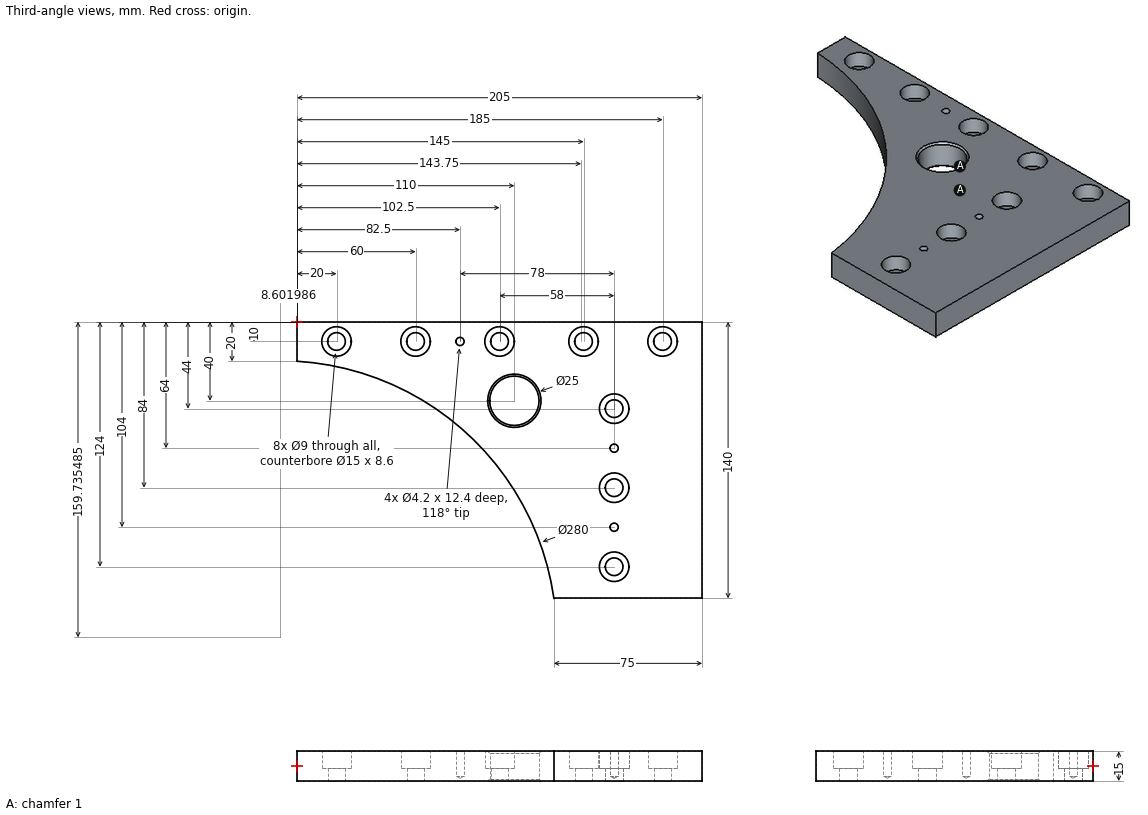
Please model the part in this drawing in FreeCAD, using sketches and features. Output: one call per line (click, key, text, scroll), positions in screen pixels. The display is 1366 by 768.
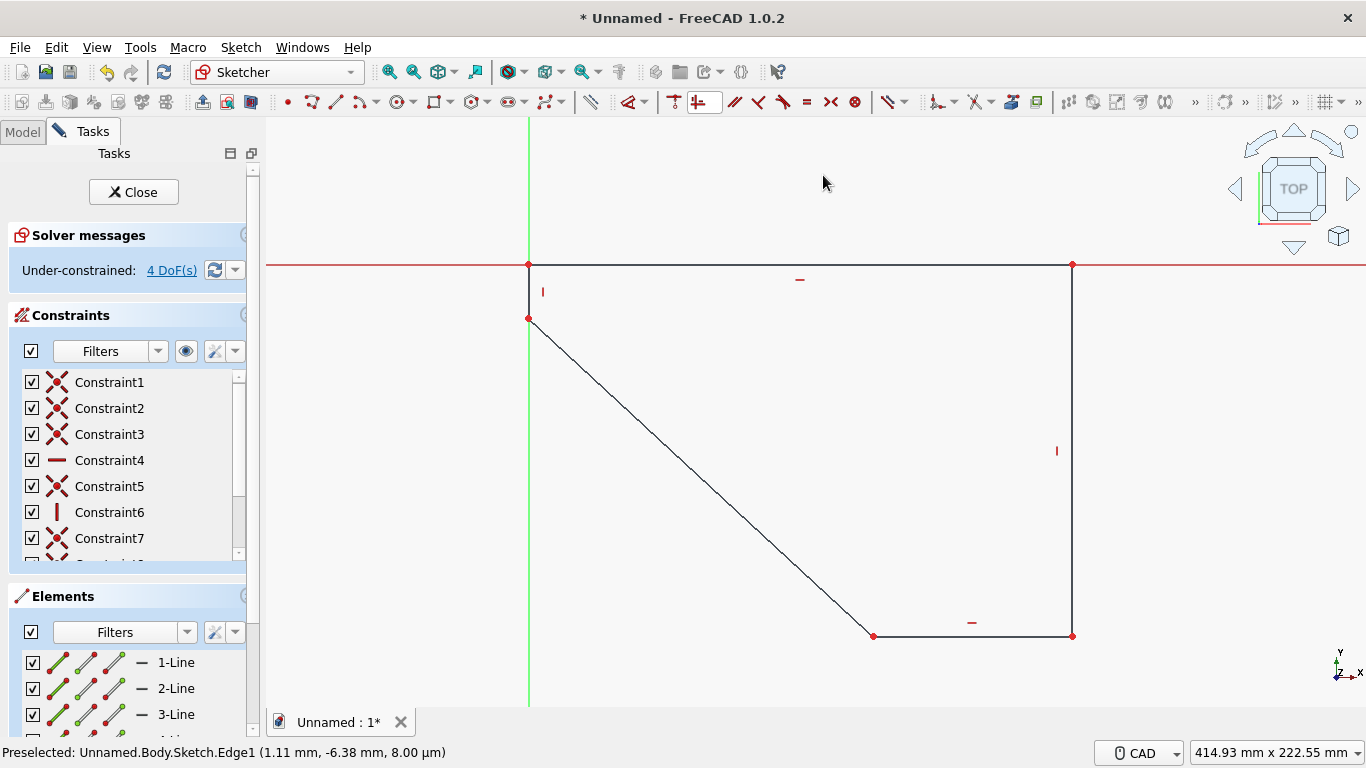
click(529, 281)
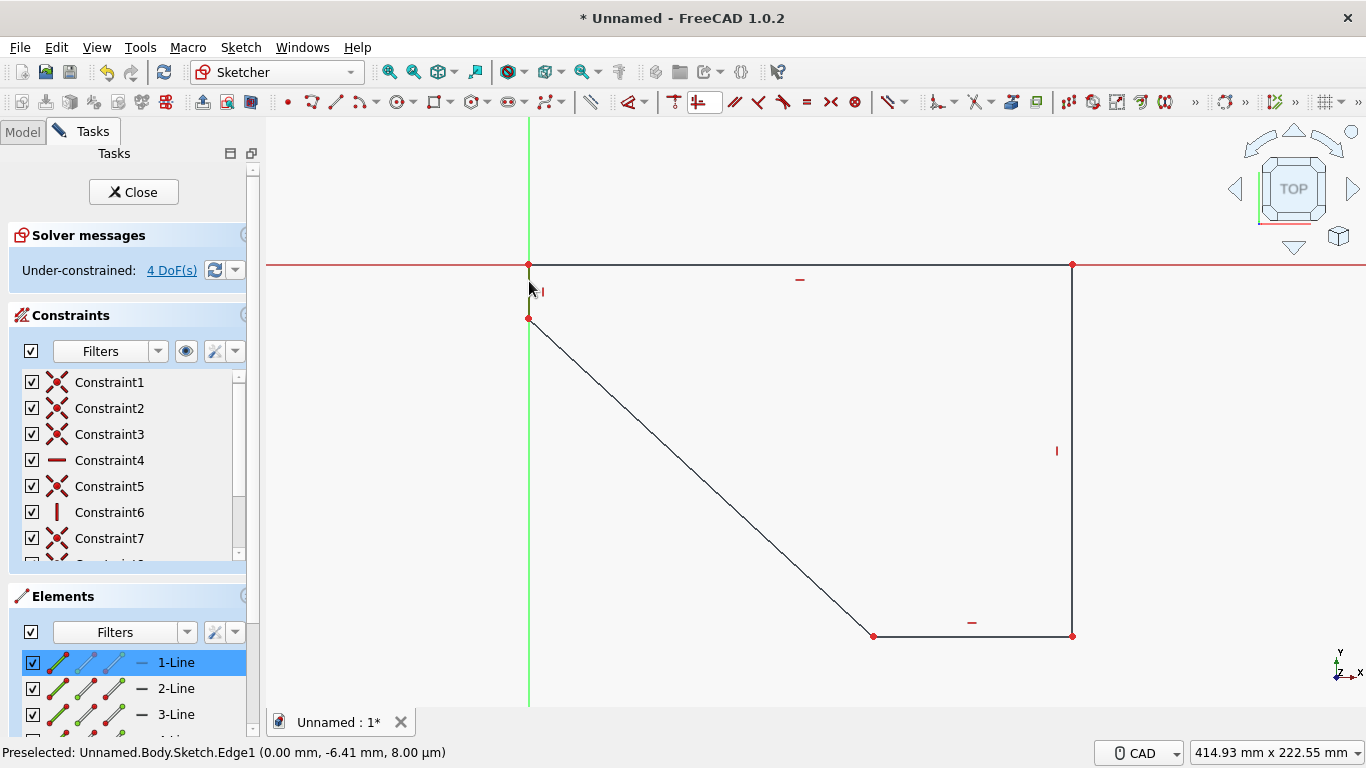
click(646, 102)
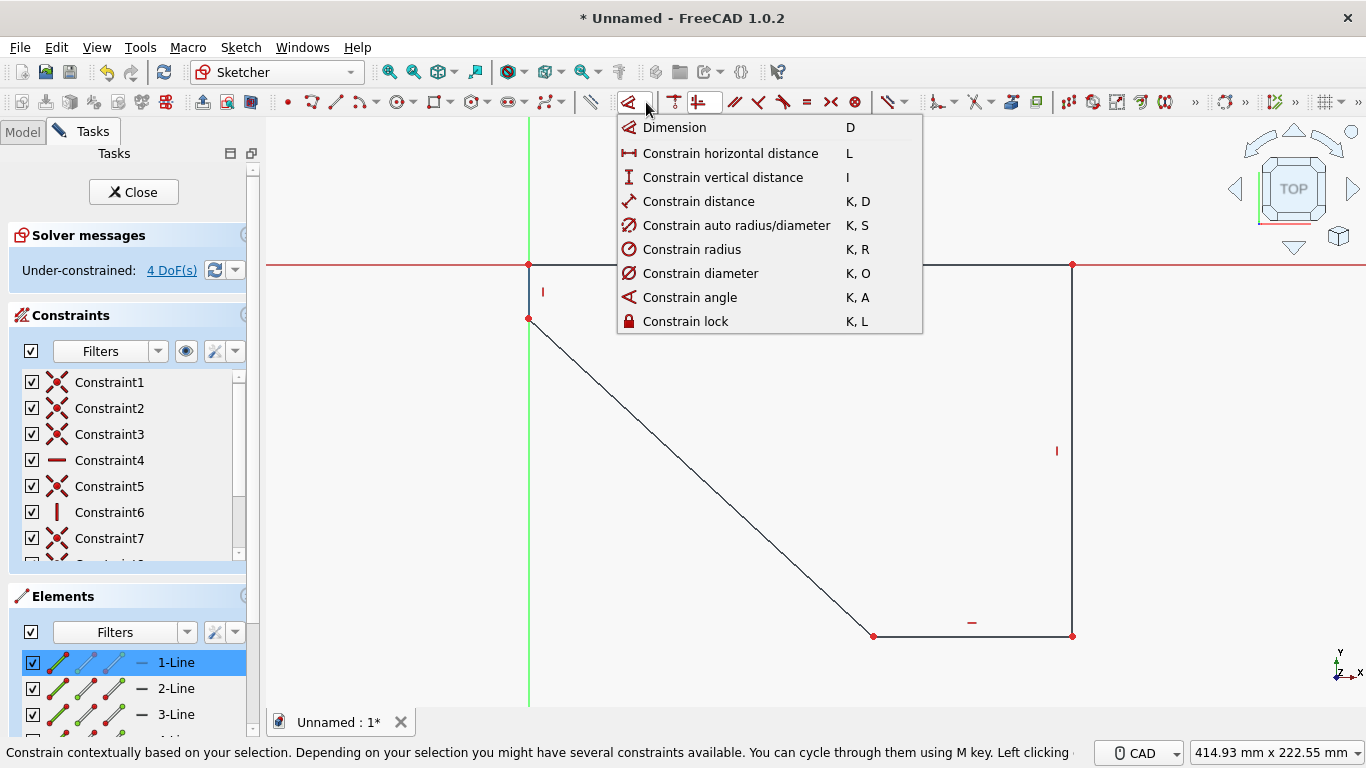
click(770, 177)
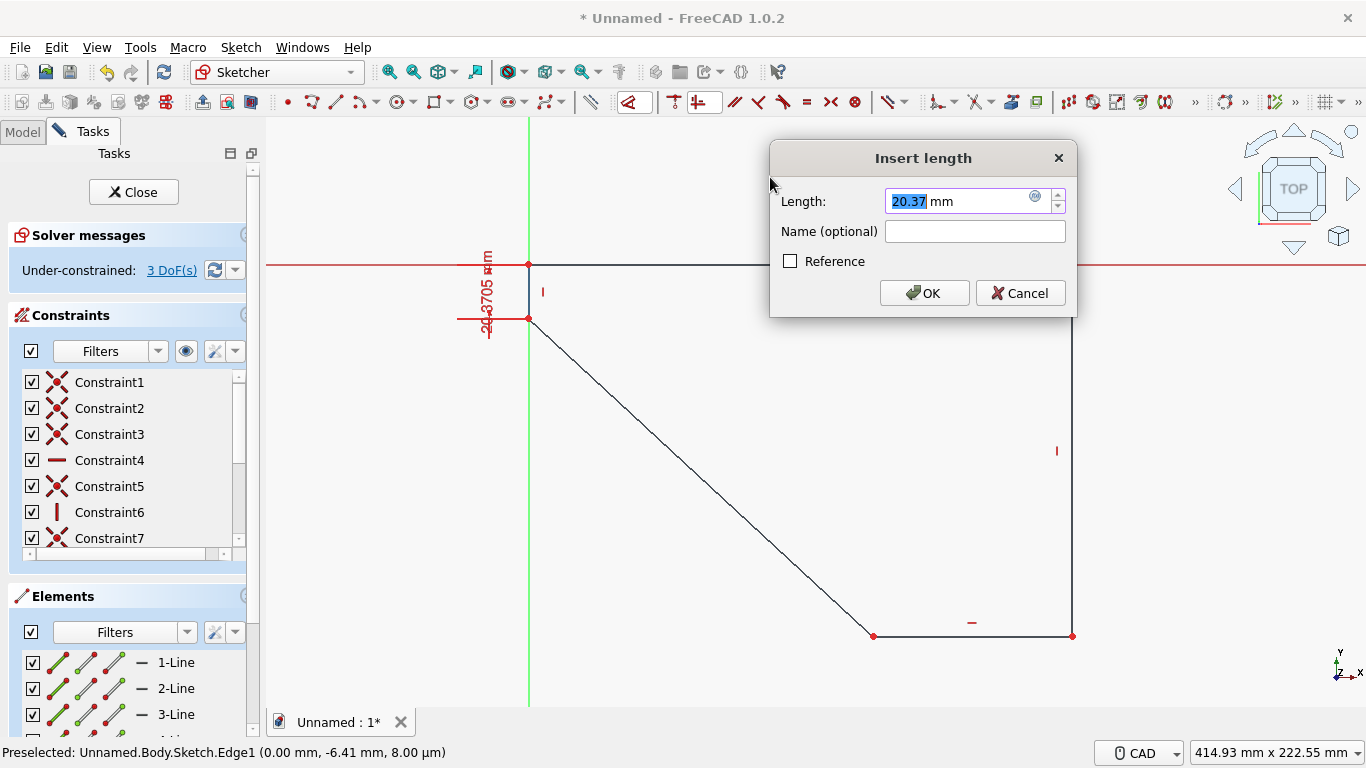
text(20)
key(Return)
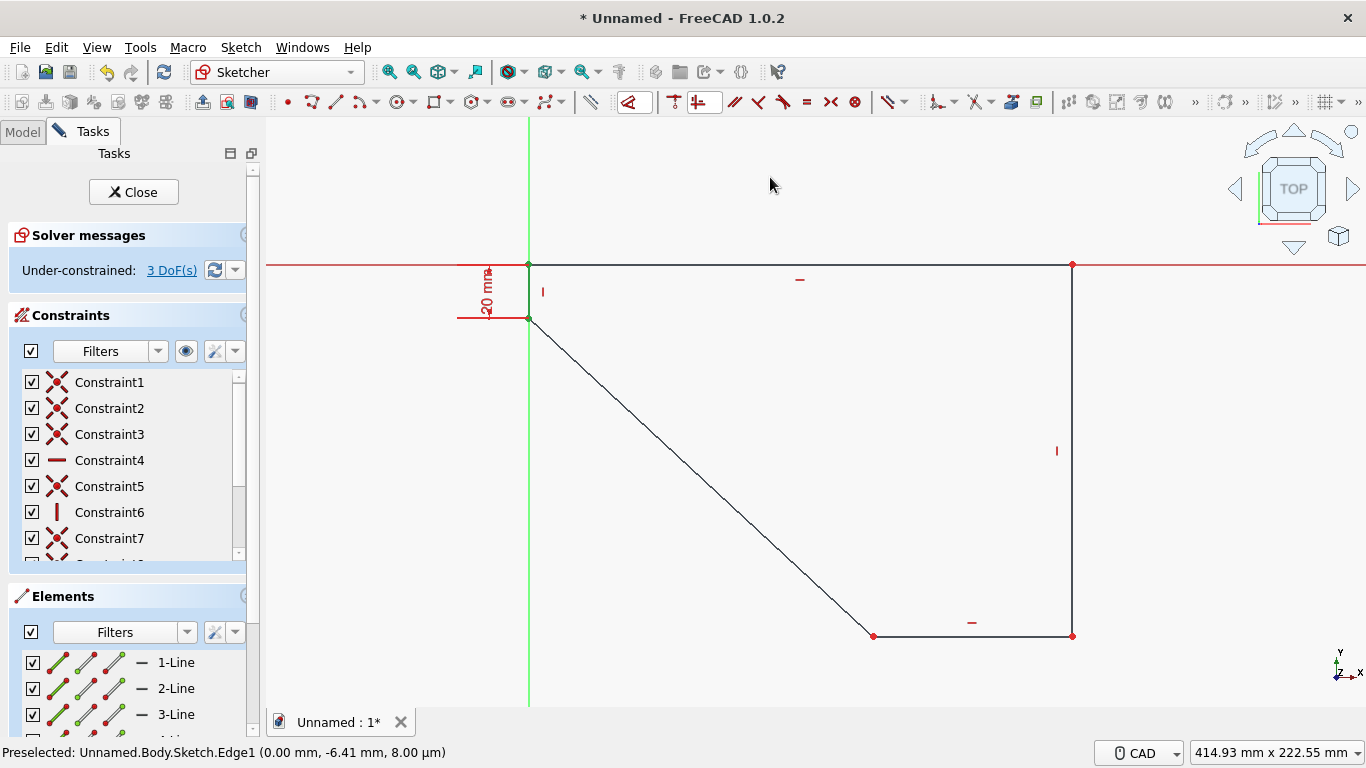
click(933, 637)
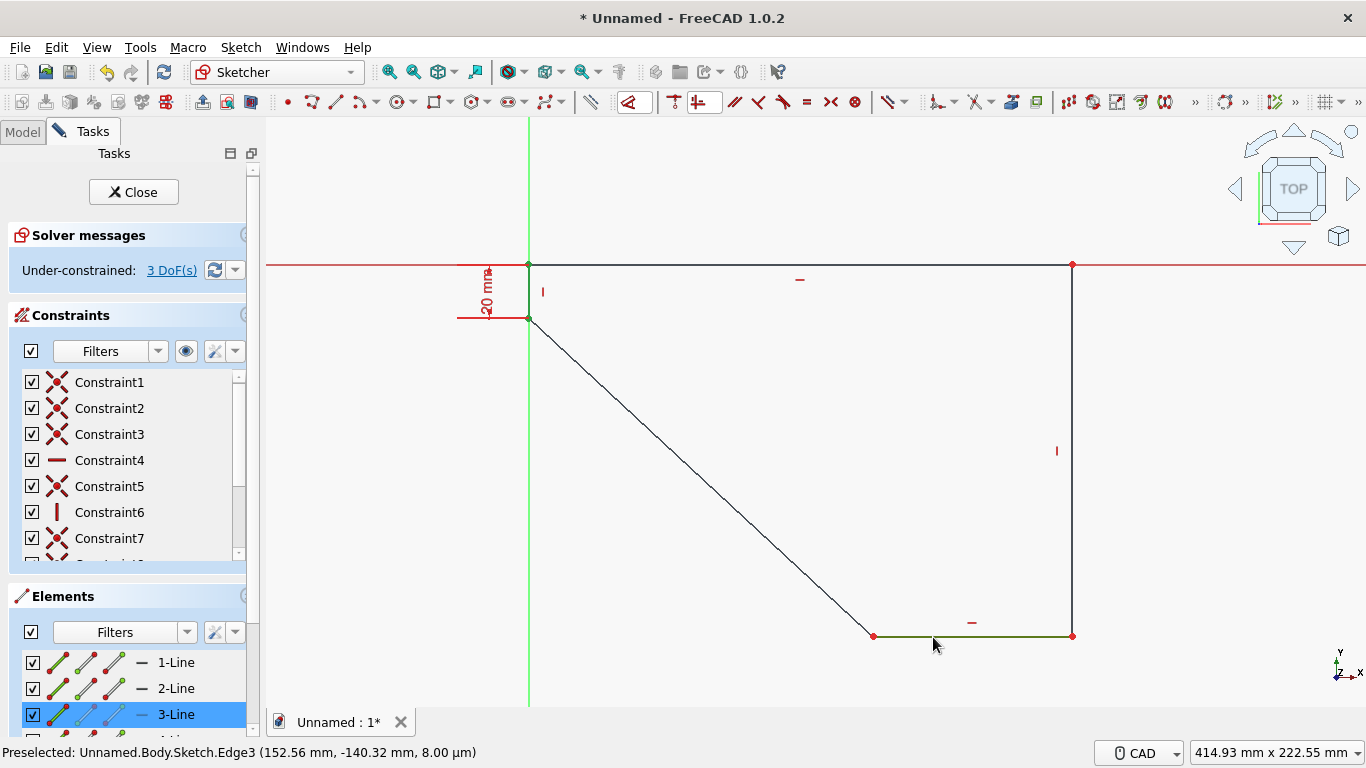
click(646, 102)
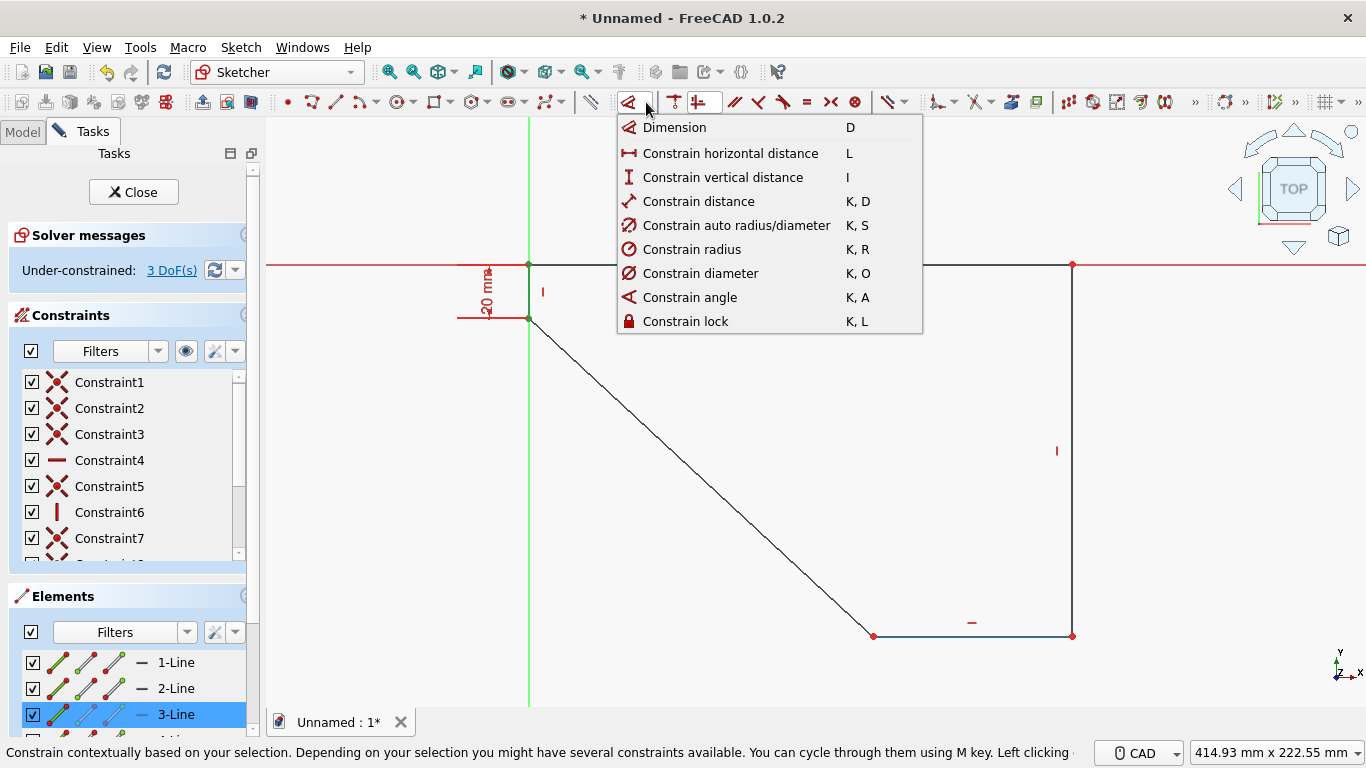
click(770, 153)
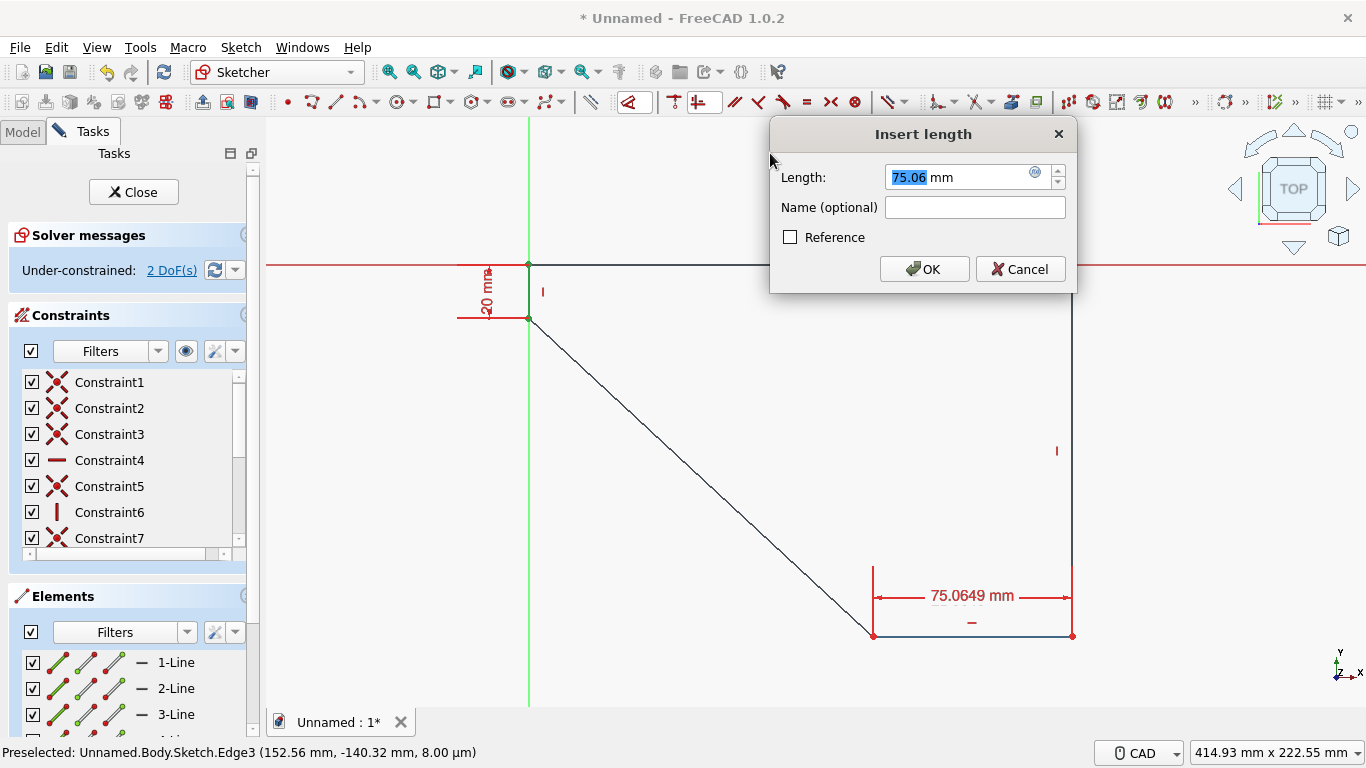
text(75)
key(Return)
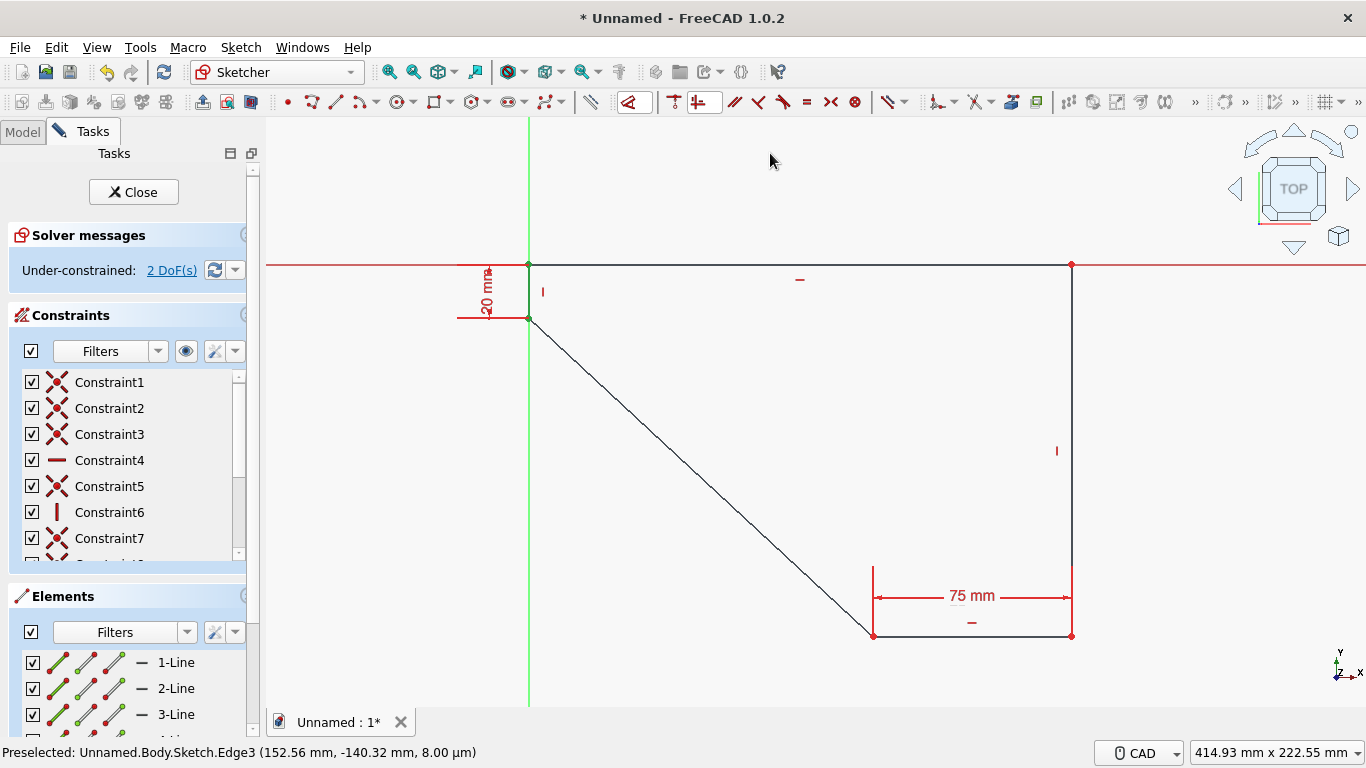
click(1072, 525)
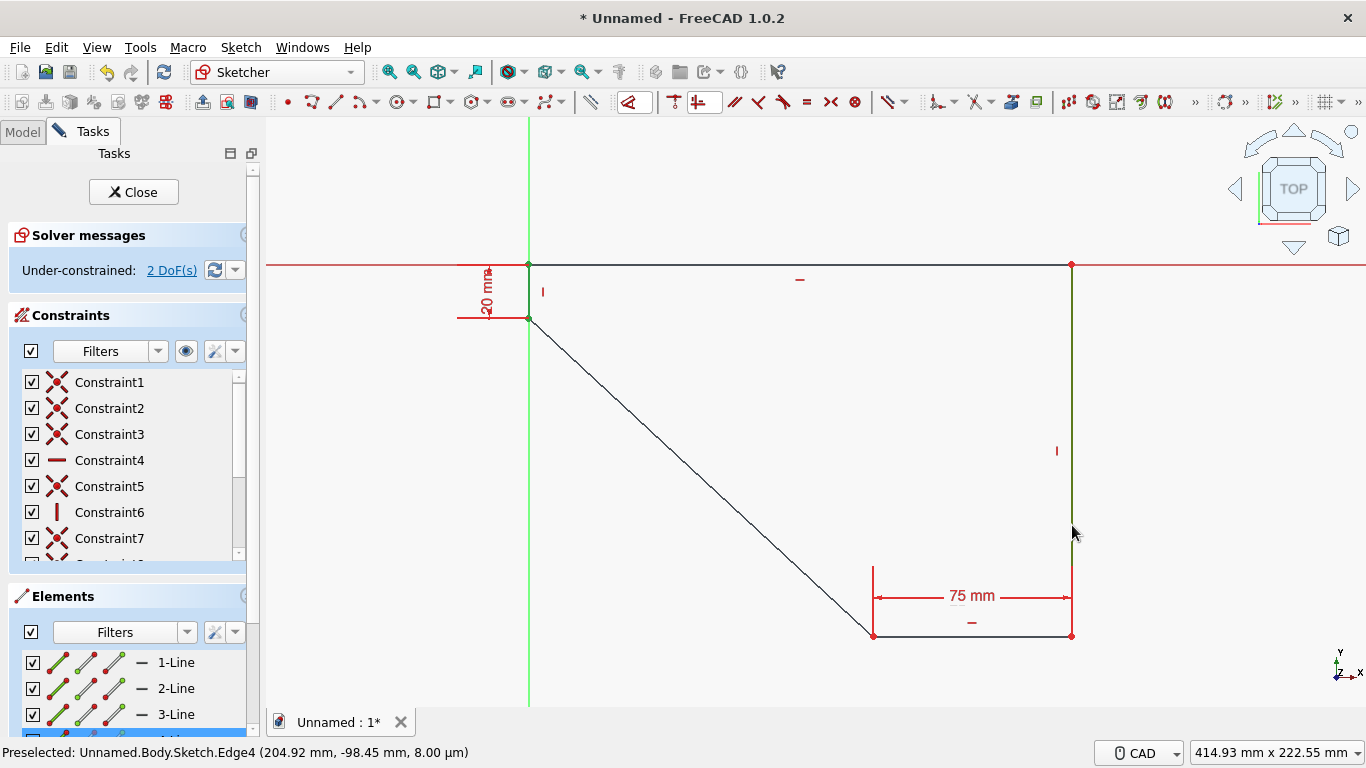
key(i)